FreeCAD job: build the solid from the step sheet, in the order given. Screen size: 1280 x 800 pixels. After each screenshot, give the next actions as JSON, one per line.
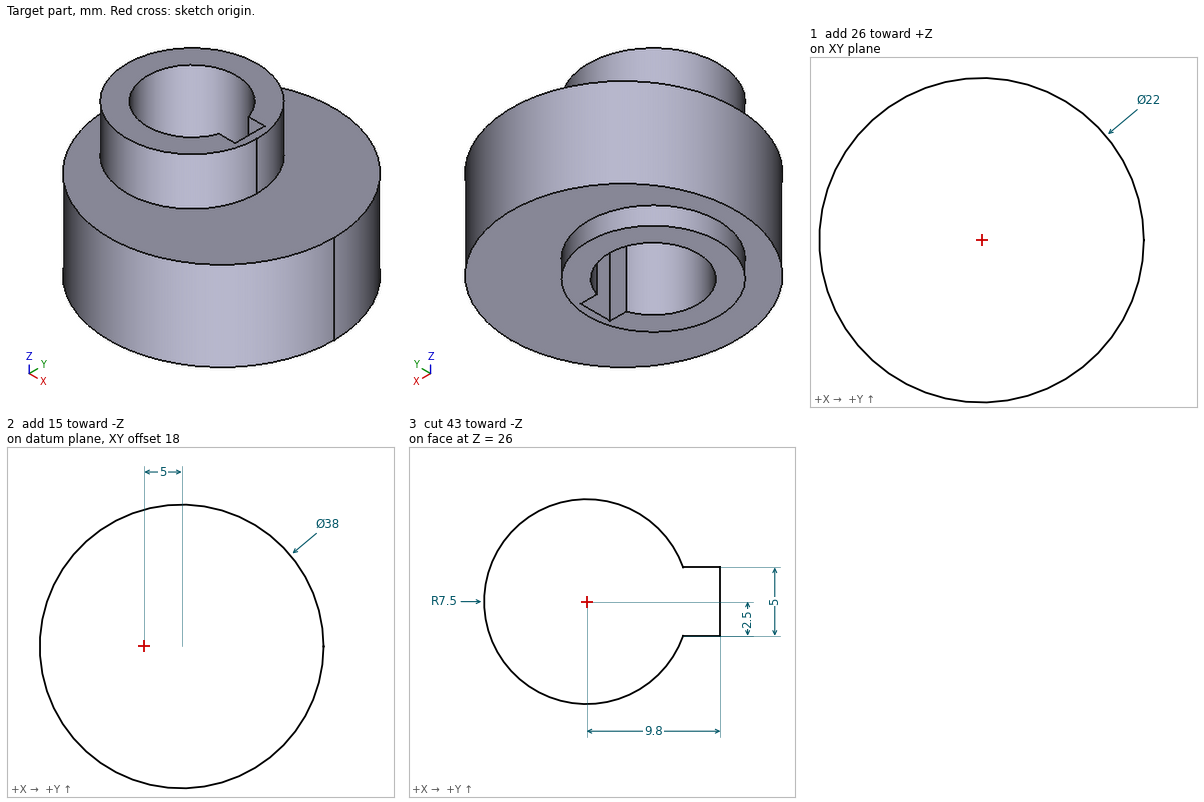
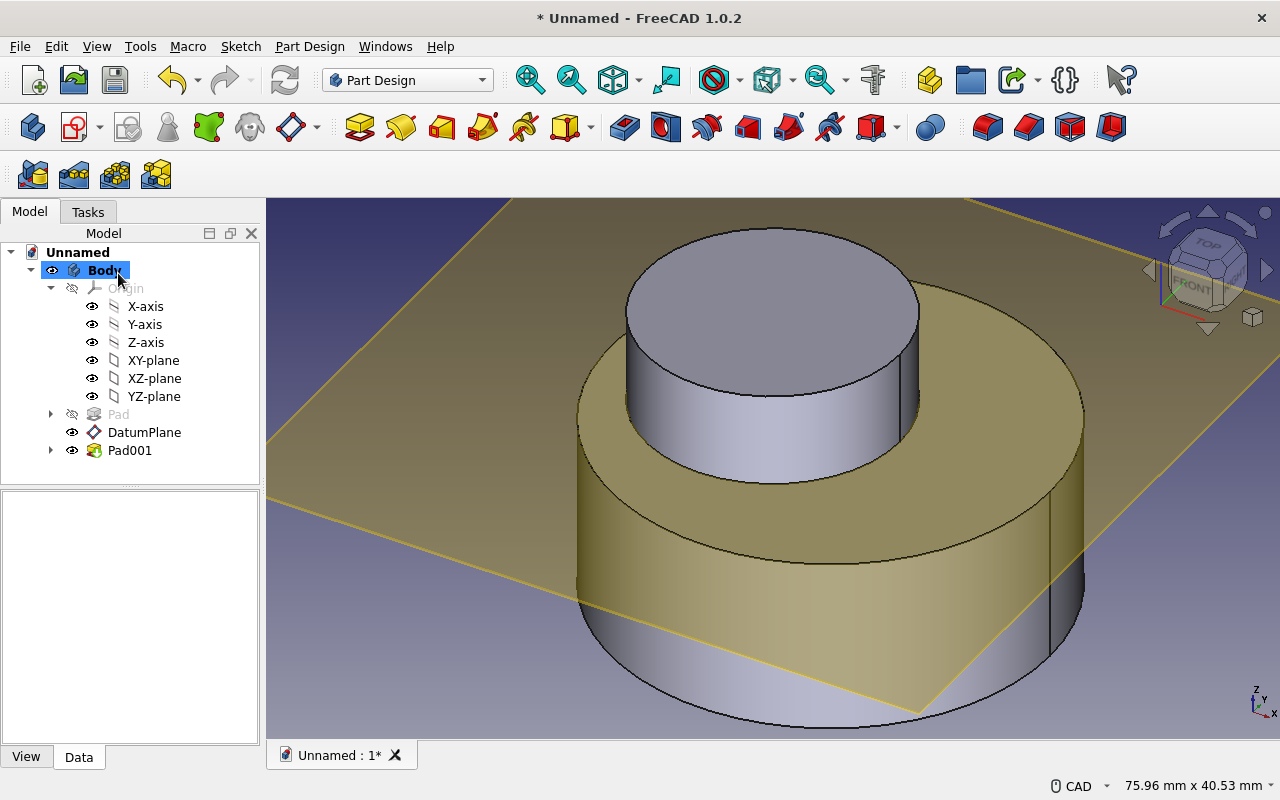
{"action": "left_click", "coordinate": [117, 432]}
{"action": "key", "text": "space"}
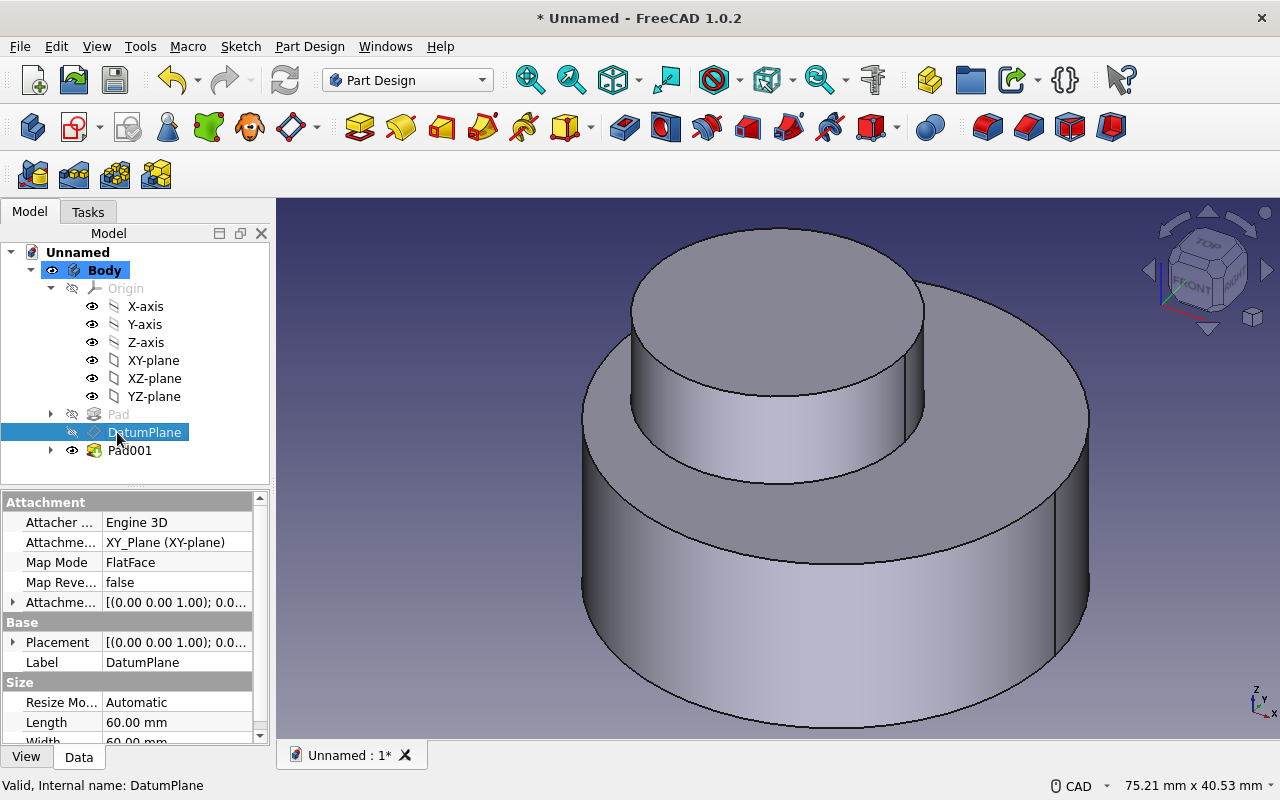
{"action": "key", "text": "v f"}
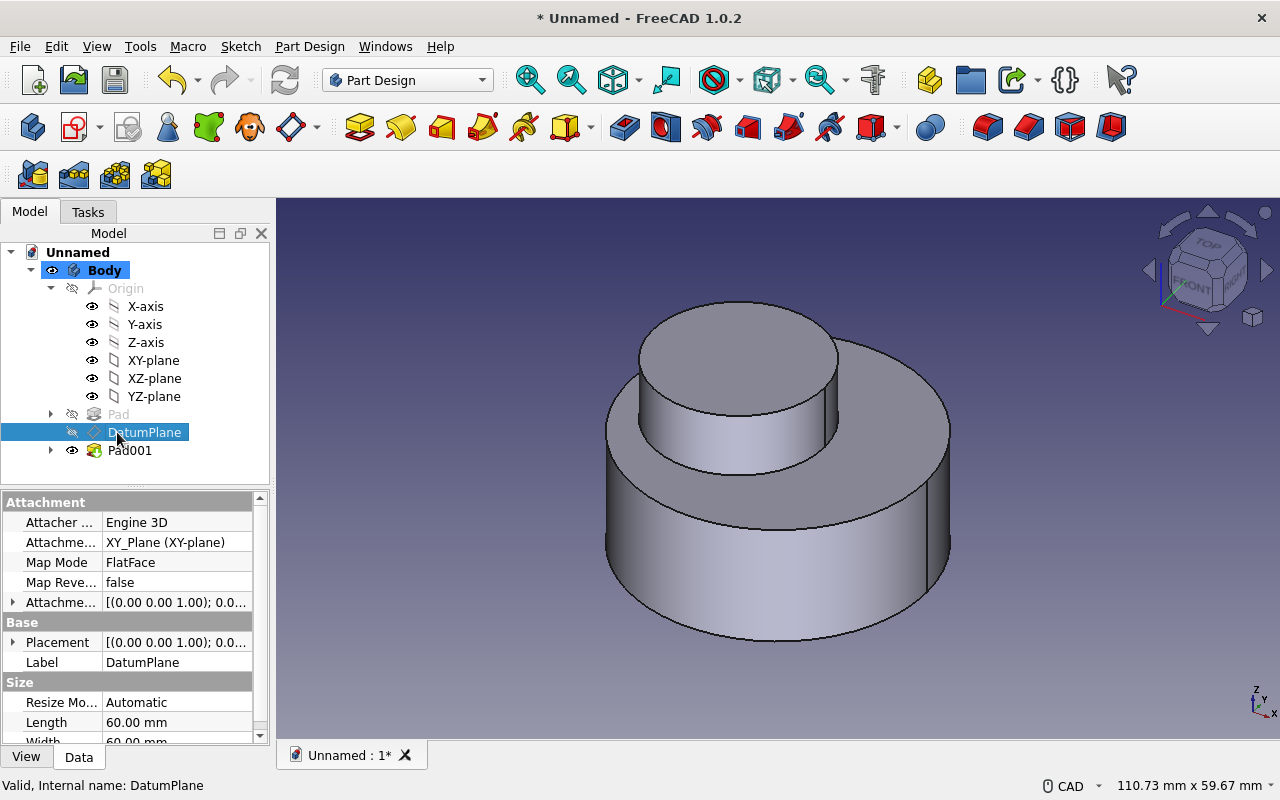
{"action": "left_click", "coordinate": [739, 358]}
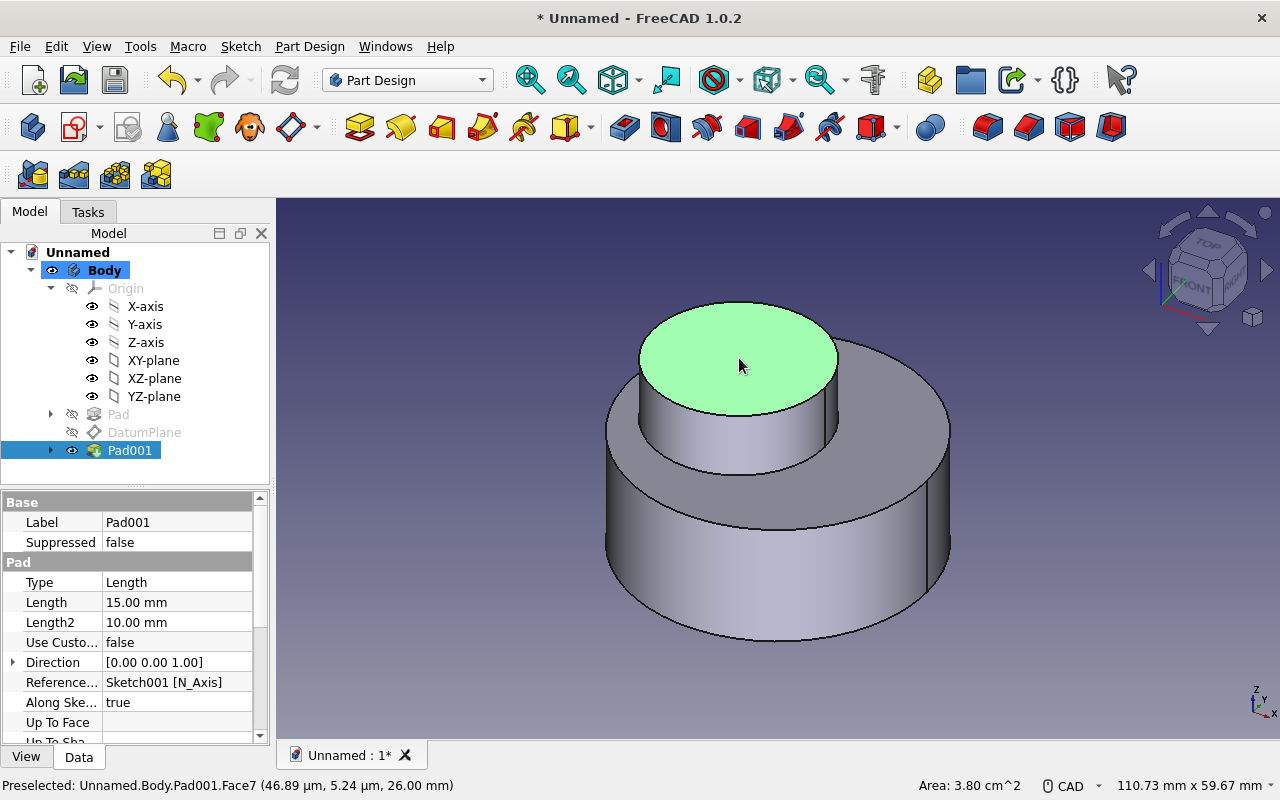
{"action": "left_click", "coordinate": [74, 128]}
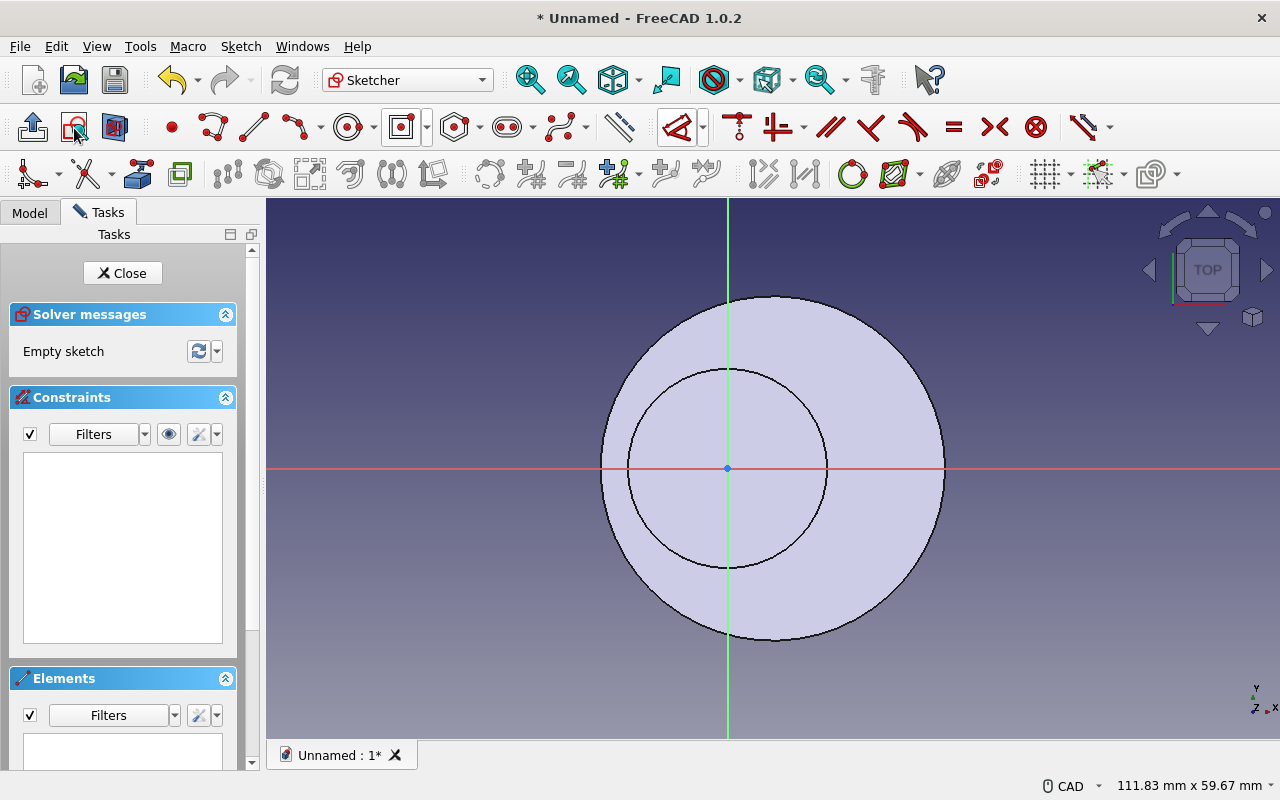
{"action": "scroll", "coordinate": [749, 468], "scroll_direction": "up", "scroll_amount": 7}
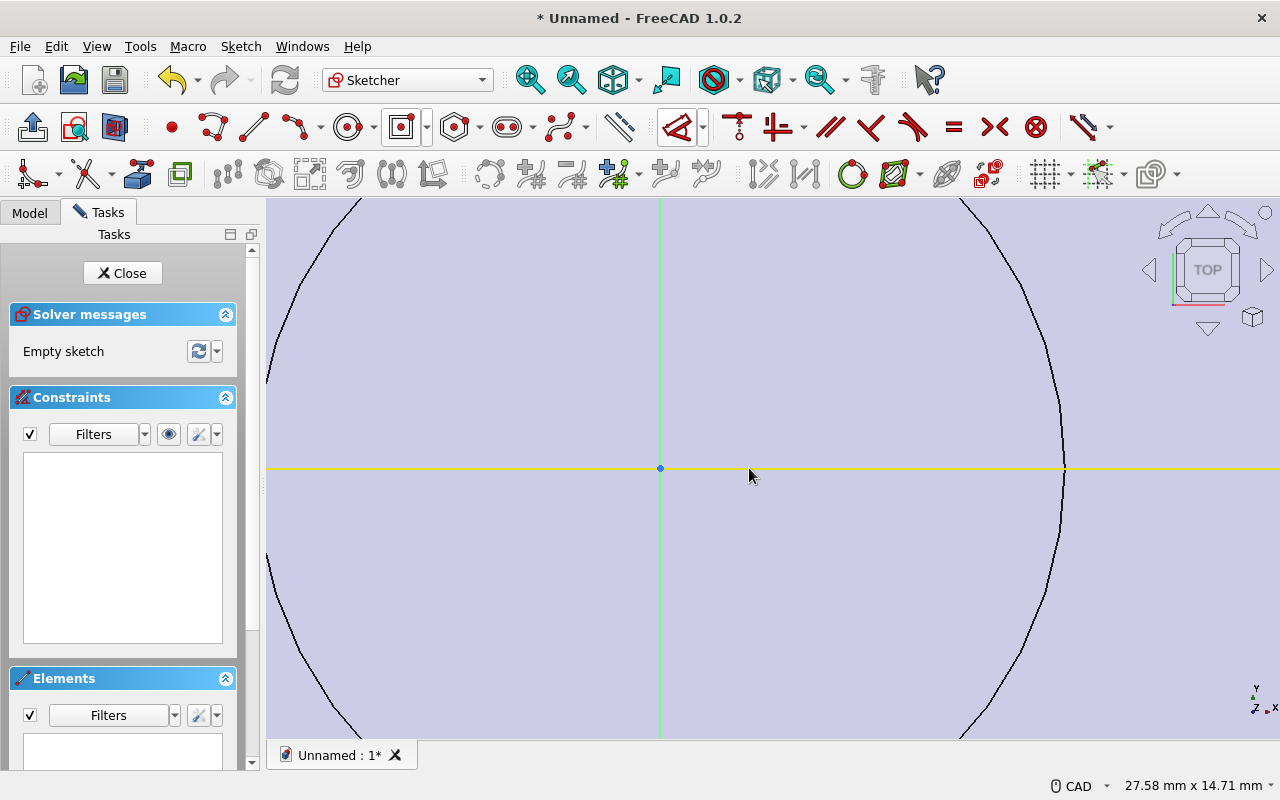
{"action": "key", "text": "g m"}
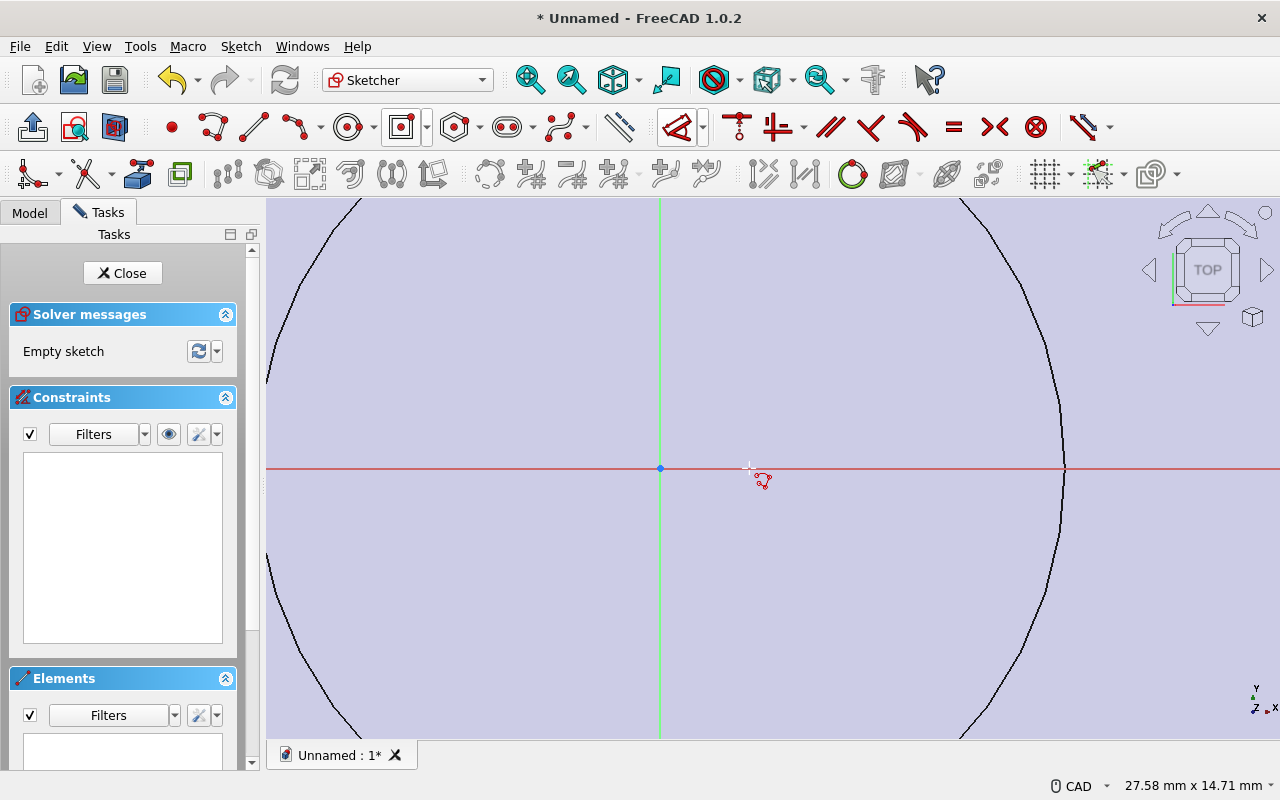
{"action": "left_click", "coordinate": [920, 560]}
{"action": "left_click", "coordinate": [1021, 560]}
{"action": "left_click", "coordinate": [1021, 377]}
{"action": "left_click", "coordinate": [920, 377]}
{"action": "right_click", "coordinate": [920, 377]}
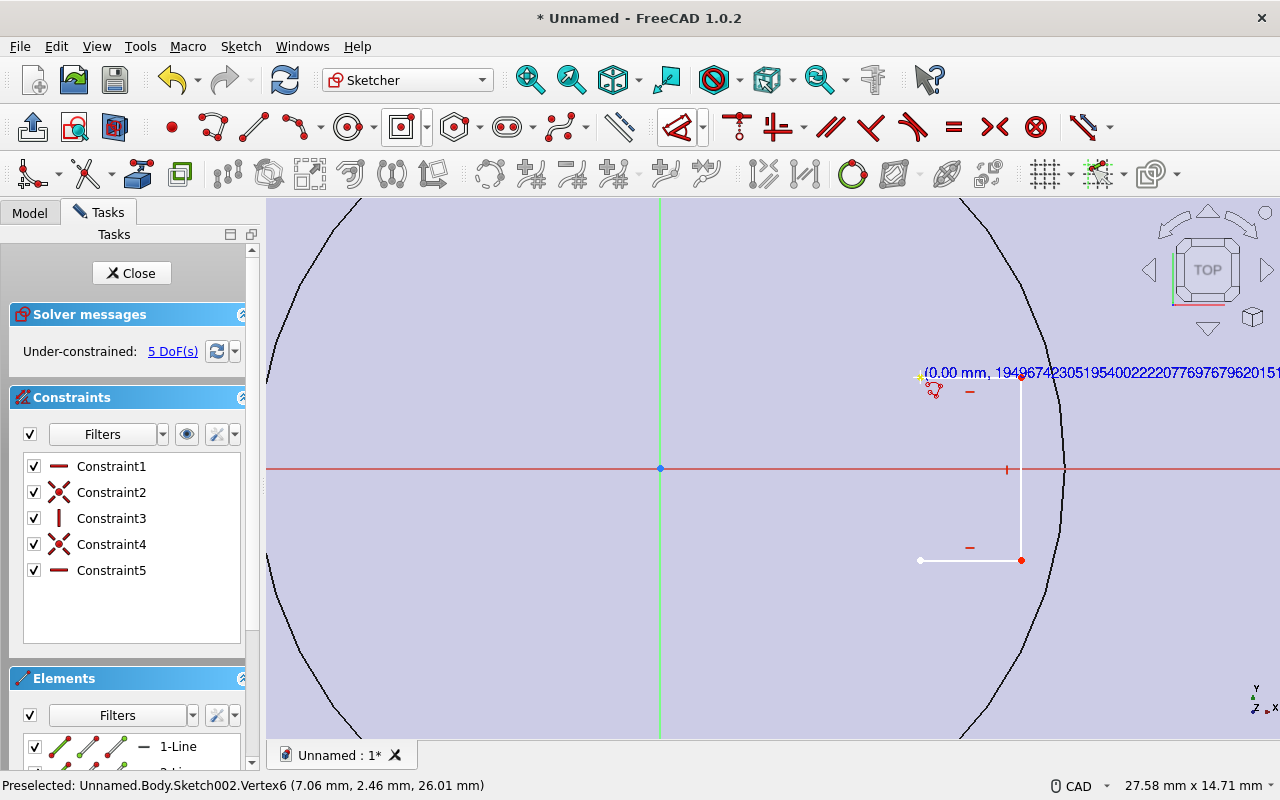
{"action": "key", "text": "g 3 a"}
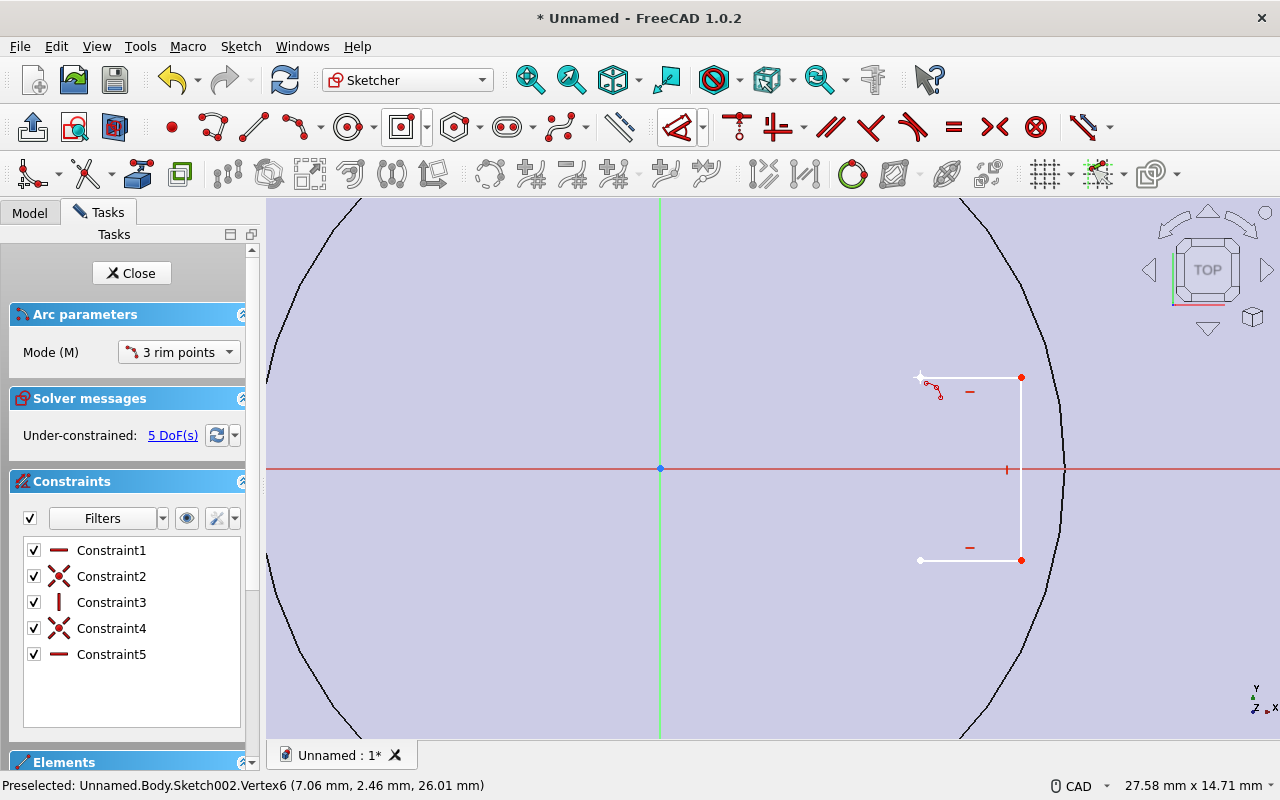
{"action": "left_click", "coordinate": [920, 378]}
{"action": "left_click", "coordinate": [920, 561]}
{"action": "left_click", "coordinate": [427, 322]}
{"action": "key", "text": "Escape"}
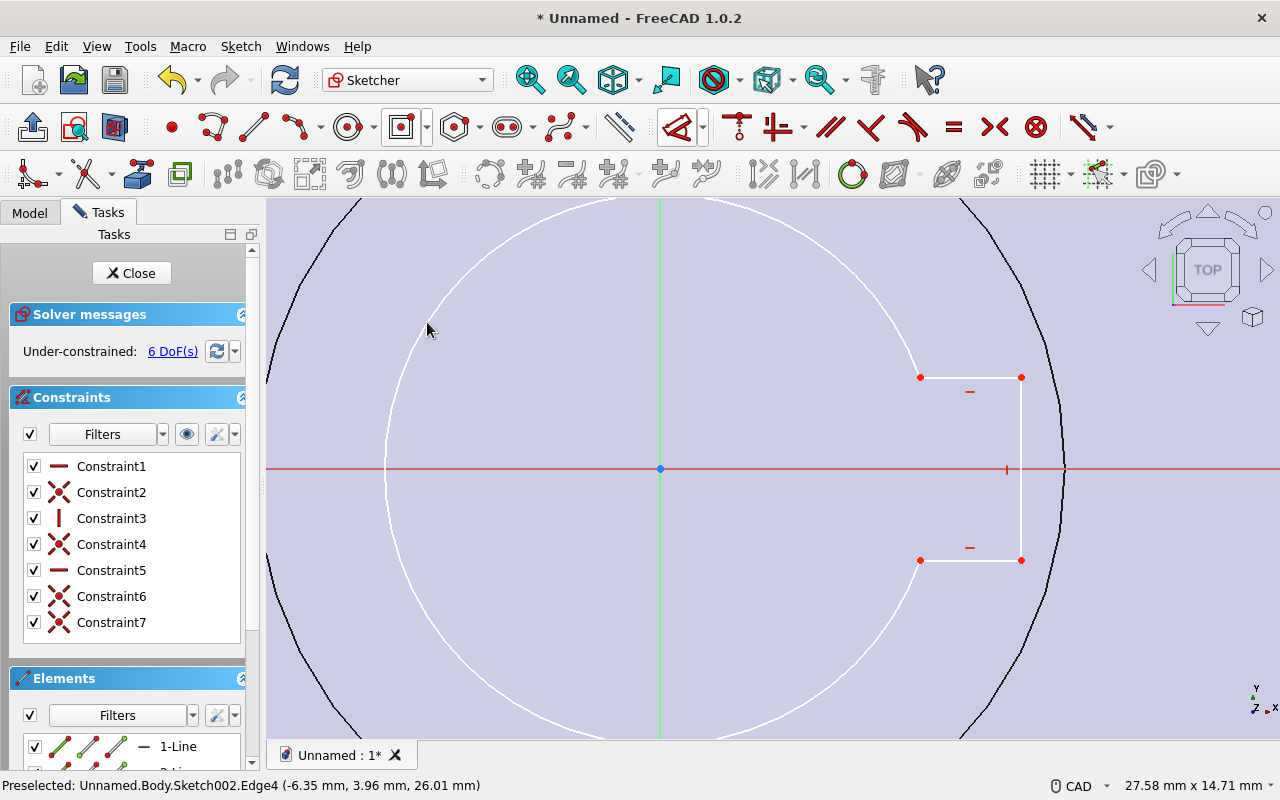
{"action": "left_click_drag", "start_coordinate": [650, 458], "coordinate": [670, 480]}